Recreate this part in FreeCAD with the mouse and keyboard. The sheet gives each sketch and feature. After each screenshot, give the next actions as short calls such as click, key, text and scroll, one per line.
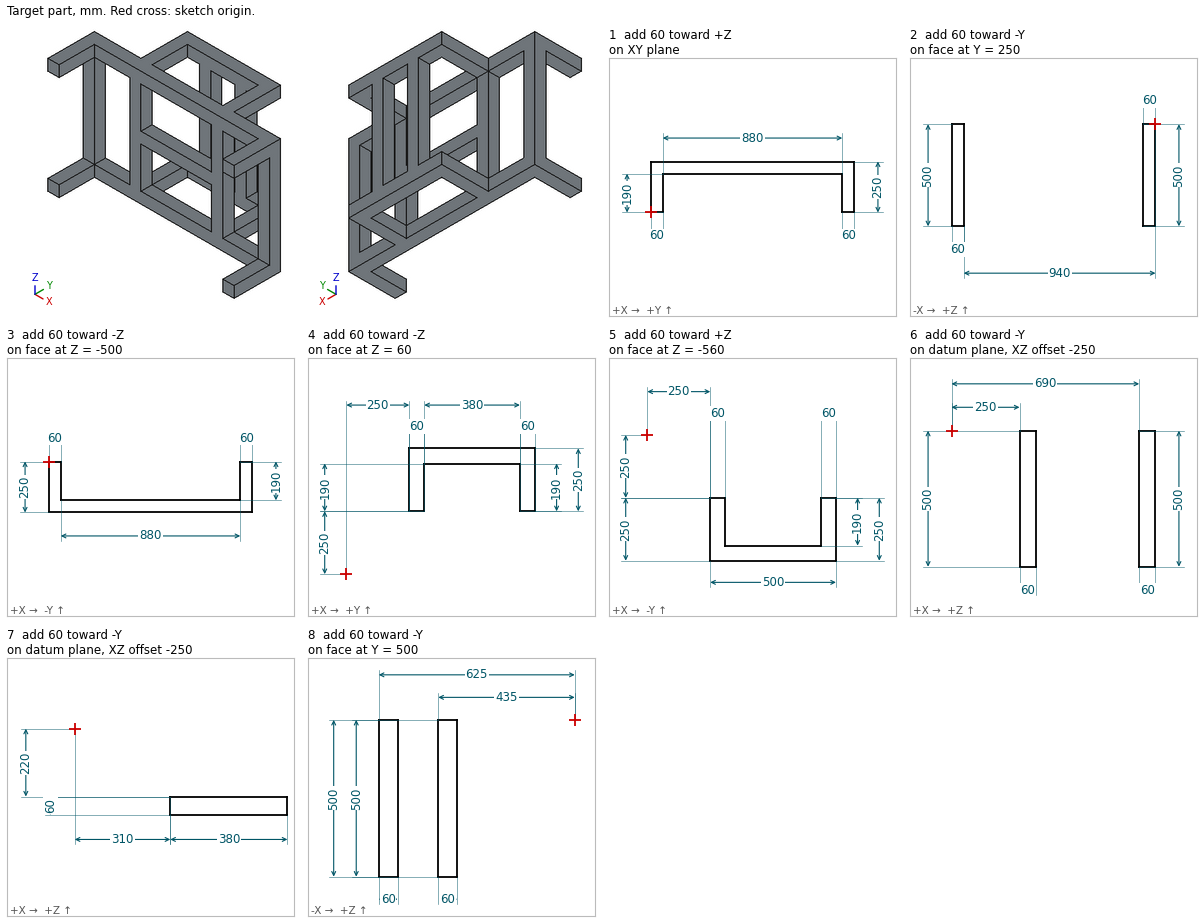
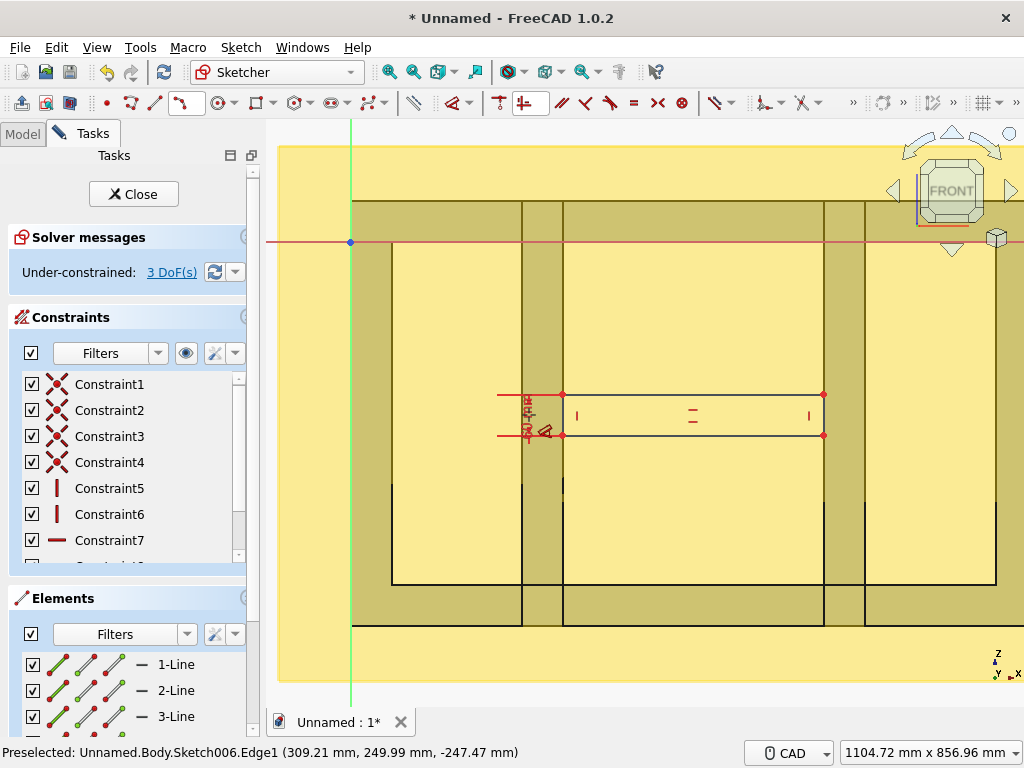
click(641, 436)
click(693, 470)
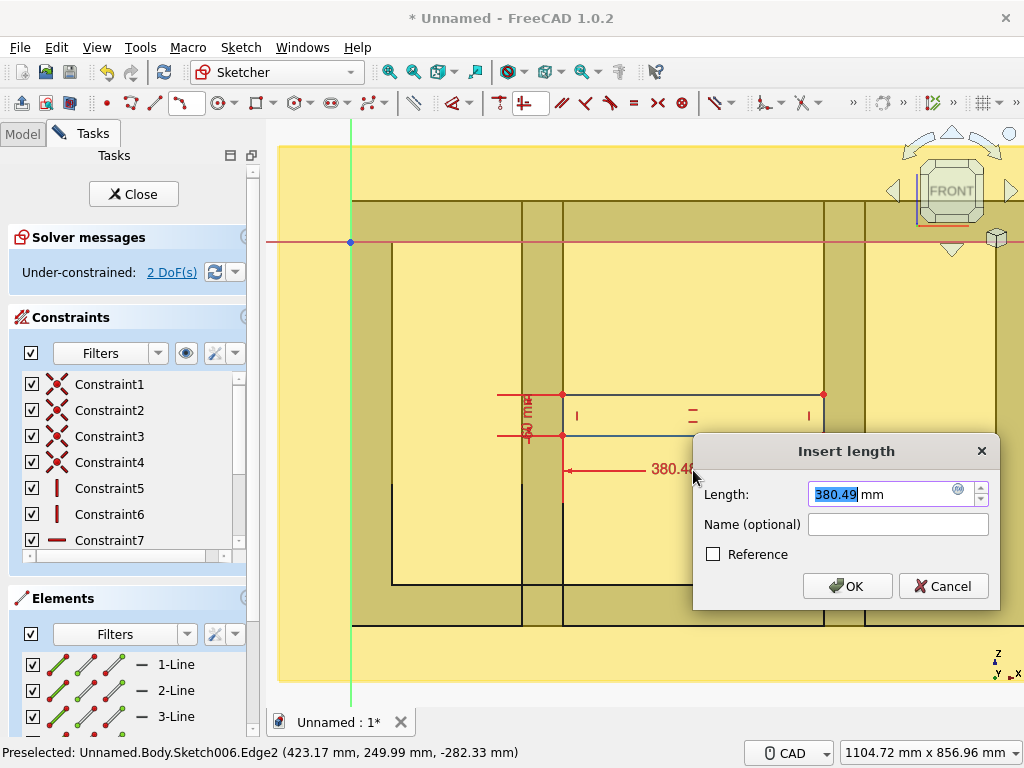
text(380)
key(Return)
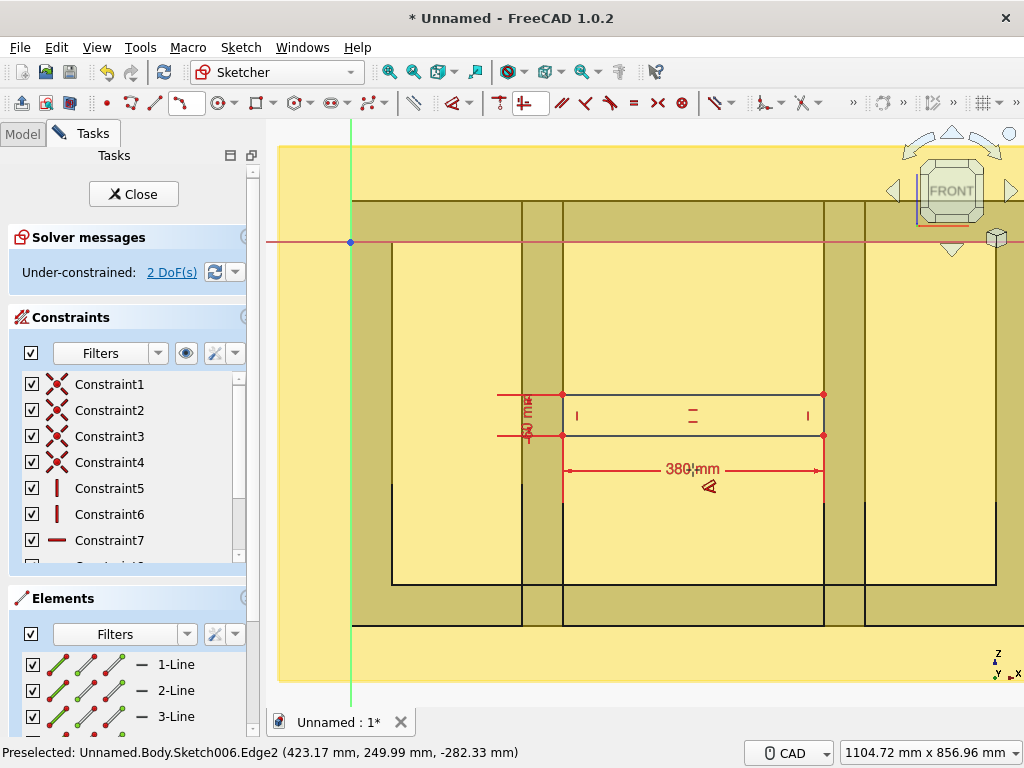
click(563, 395)
click(457, 208)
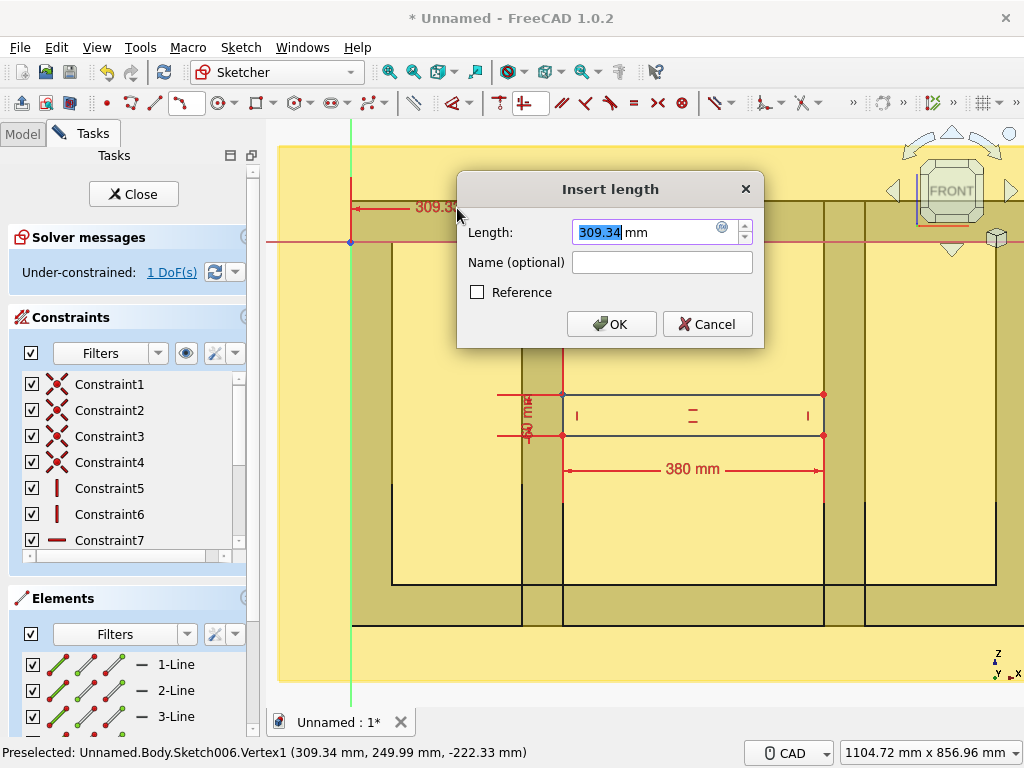
text(310)
key(Return)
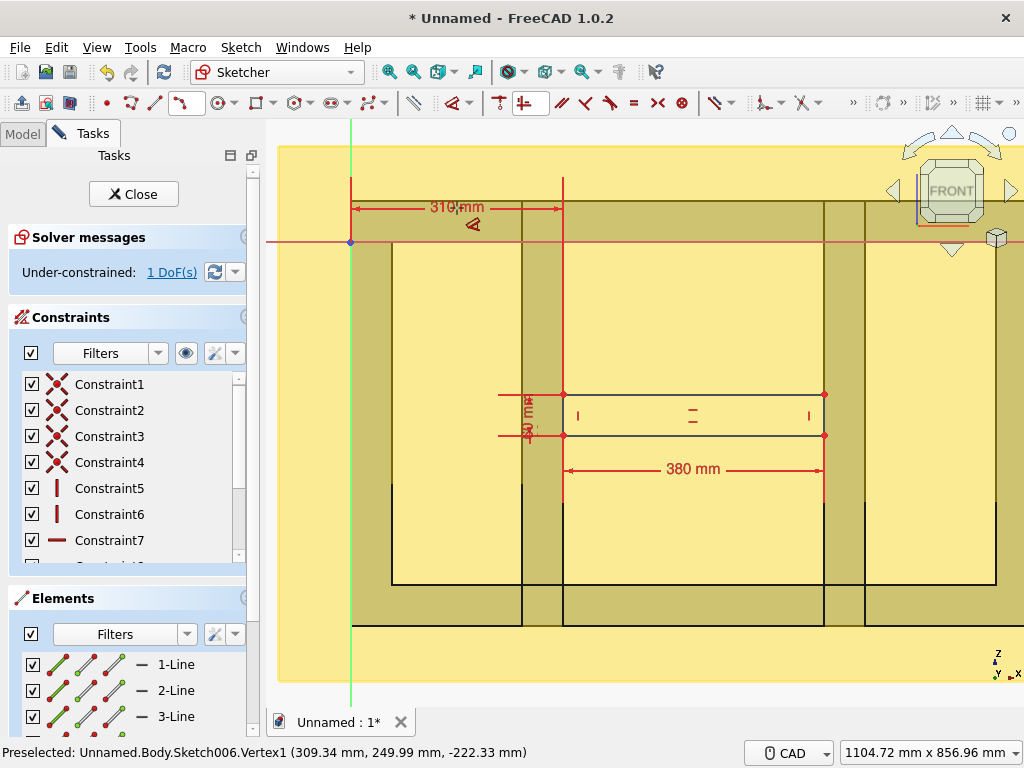
click(563, 395)
click(317, 318)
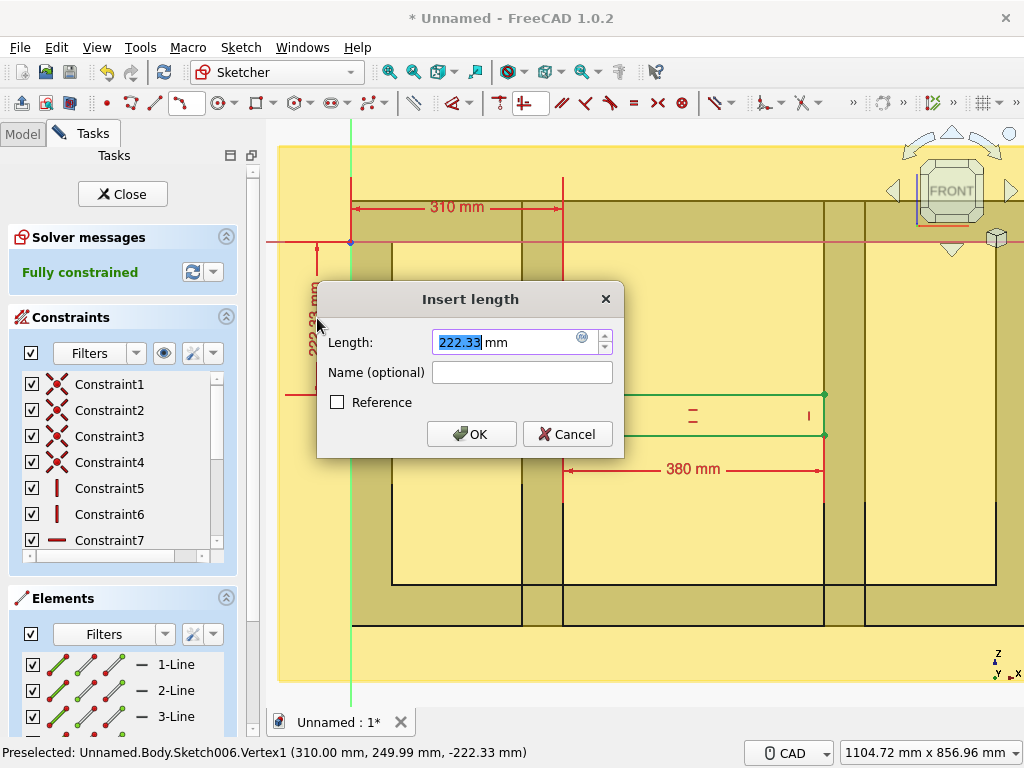
text(220)
key(Return)
key(Escape)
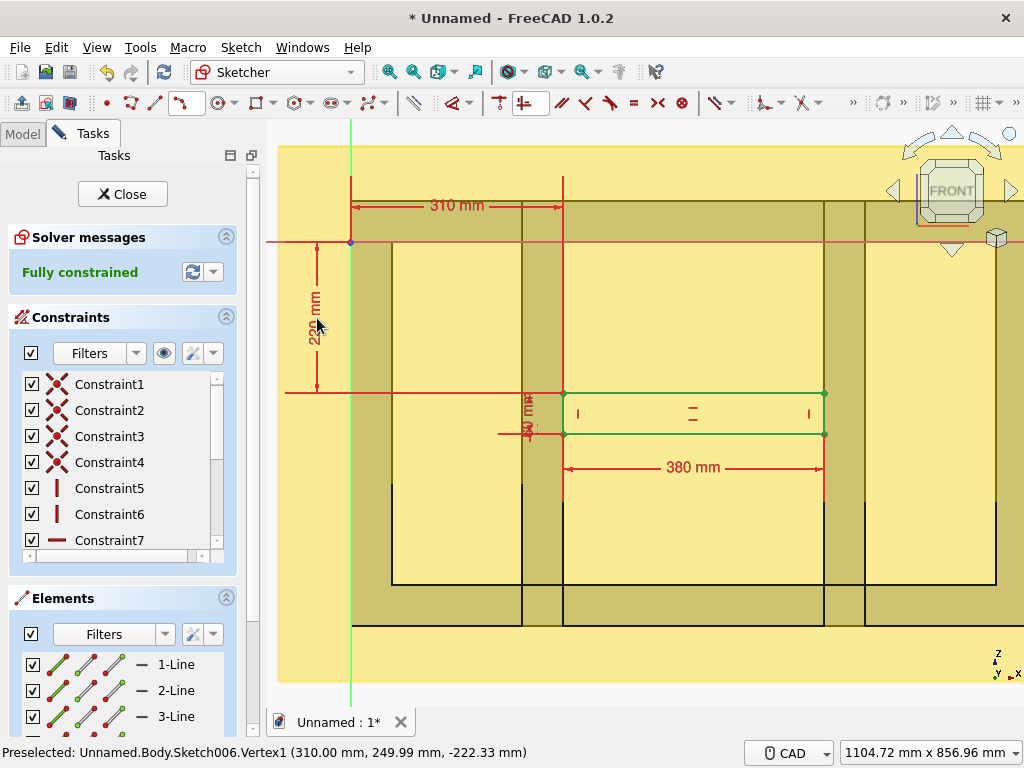
click(123, 194)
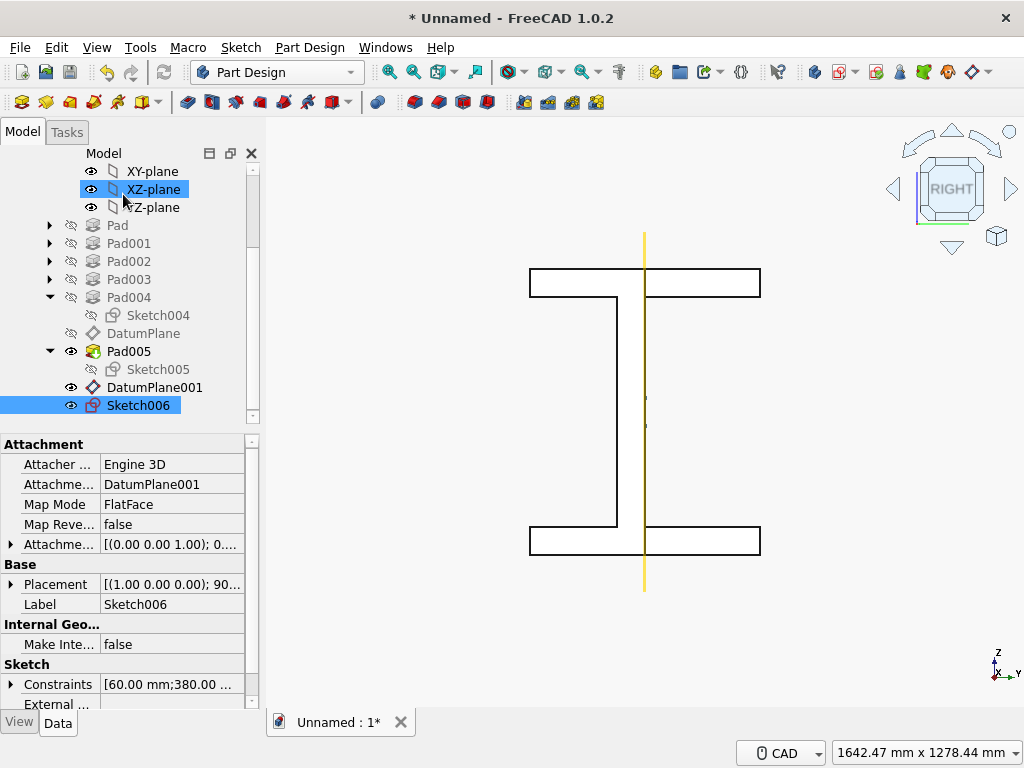
click(22, 102)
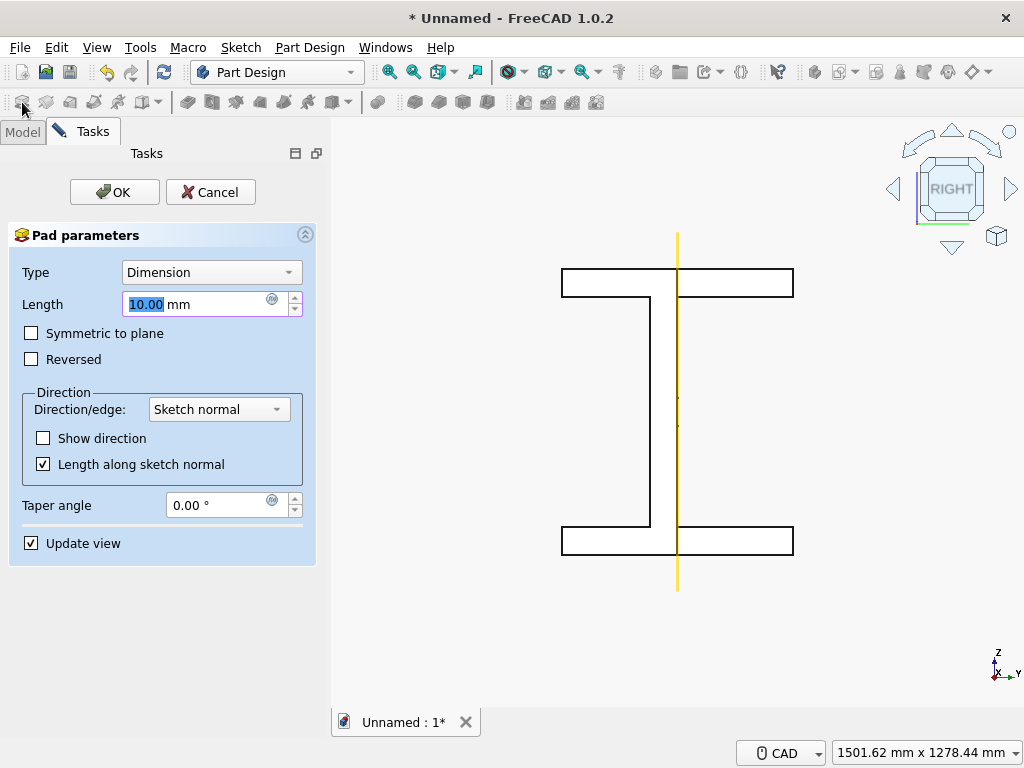
text(60)
key(Tab)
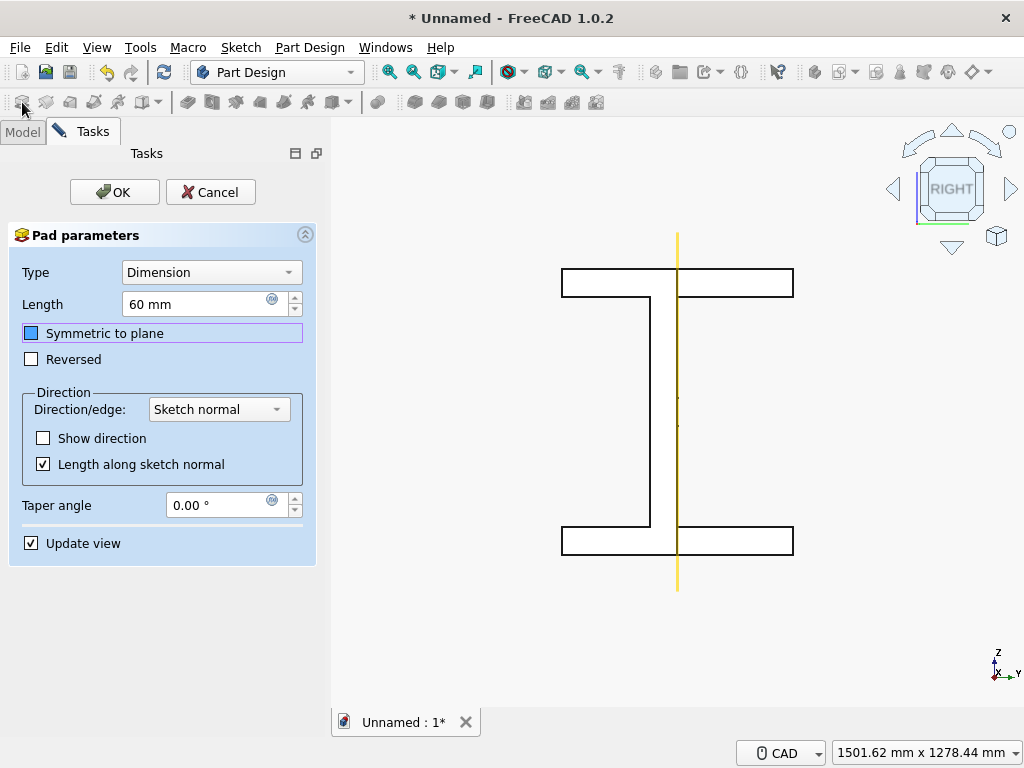
click(115, 192)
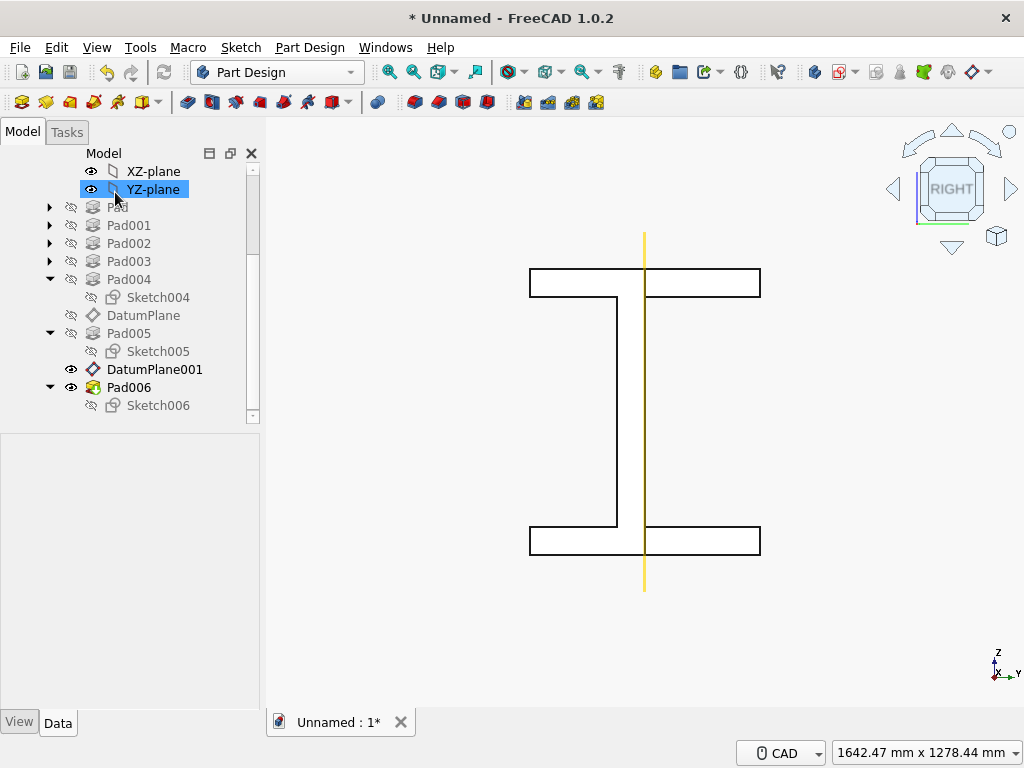
click(116, 369)
key(space)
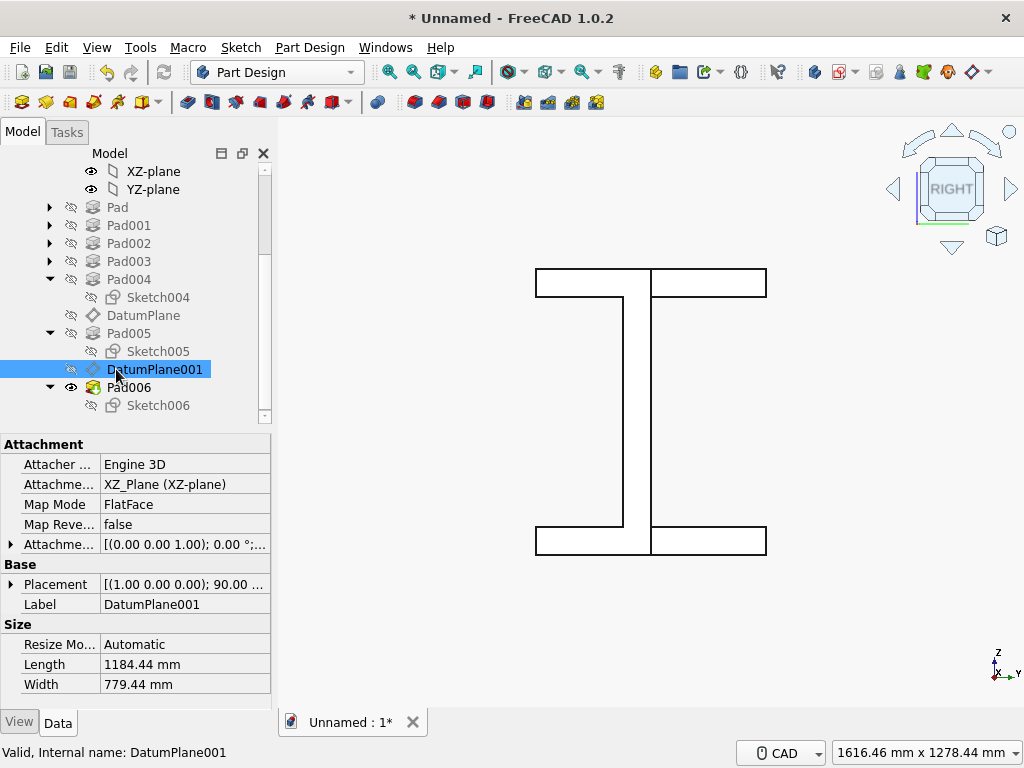
key(4)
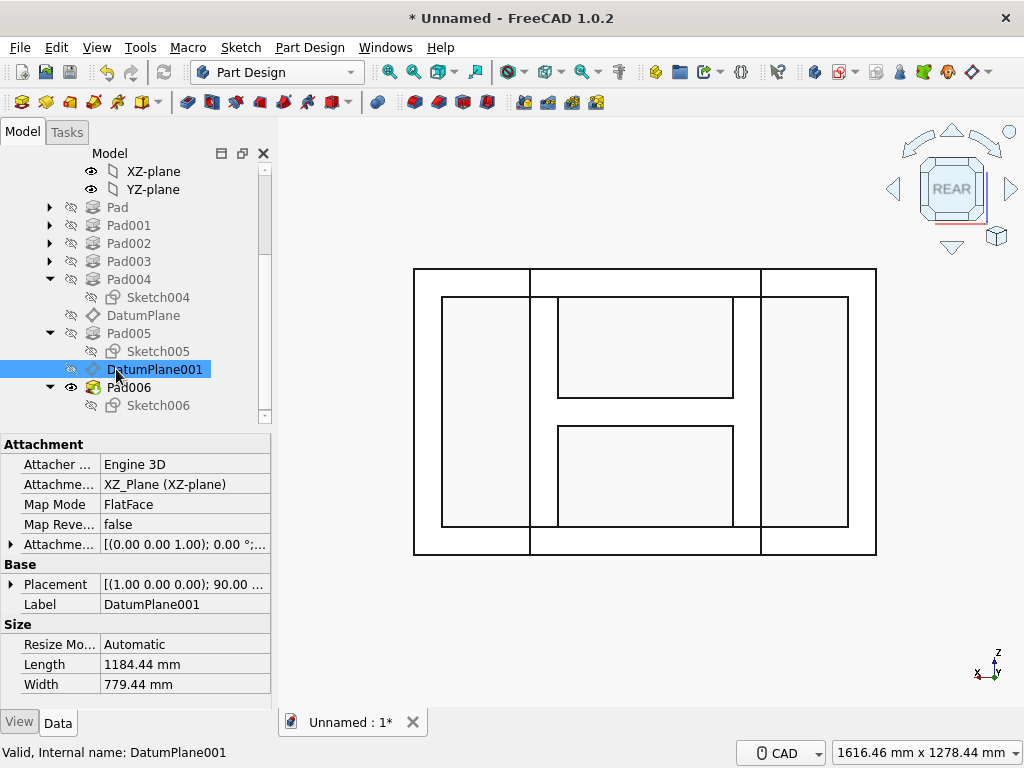
click(546, 282)